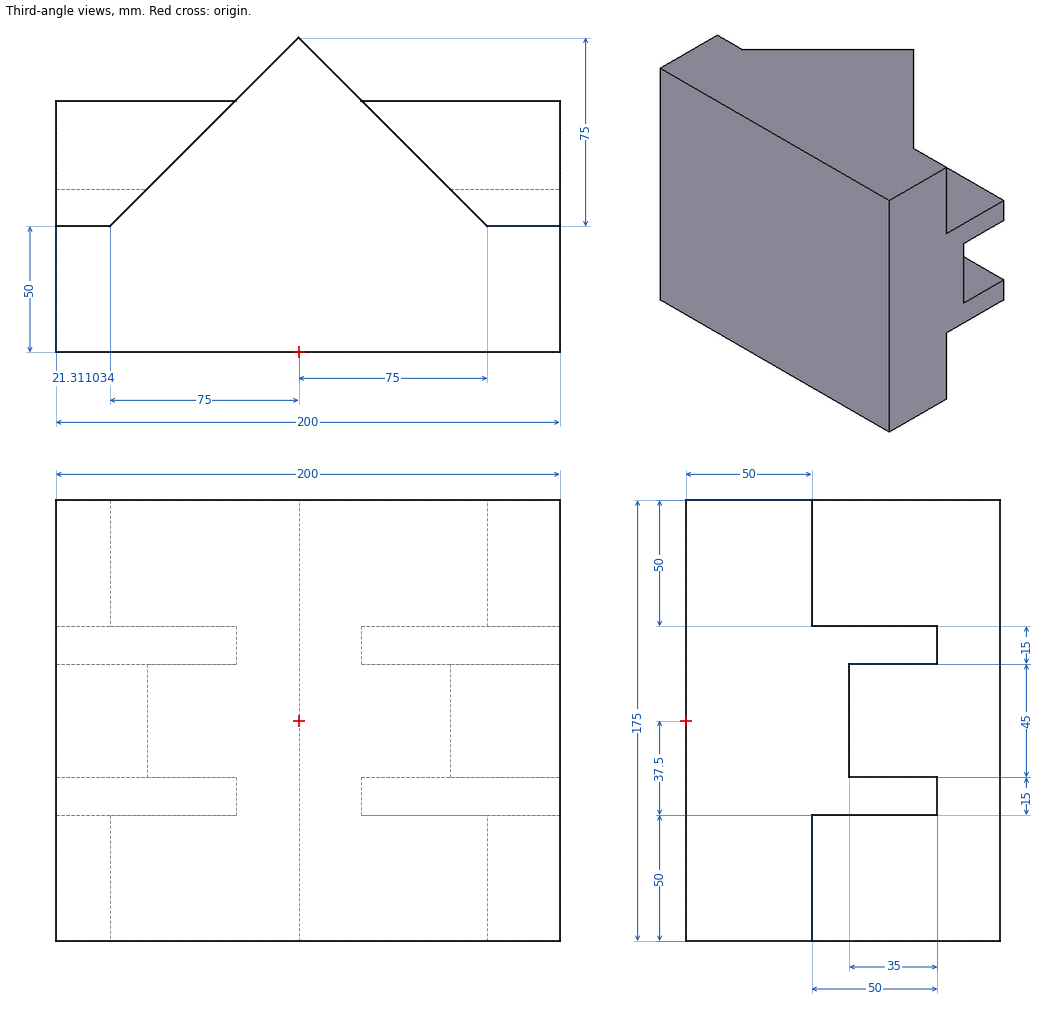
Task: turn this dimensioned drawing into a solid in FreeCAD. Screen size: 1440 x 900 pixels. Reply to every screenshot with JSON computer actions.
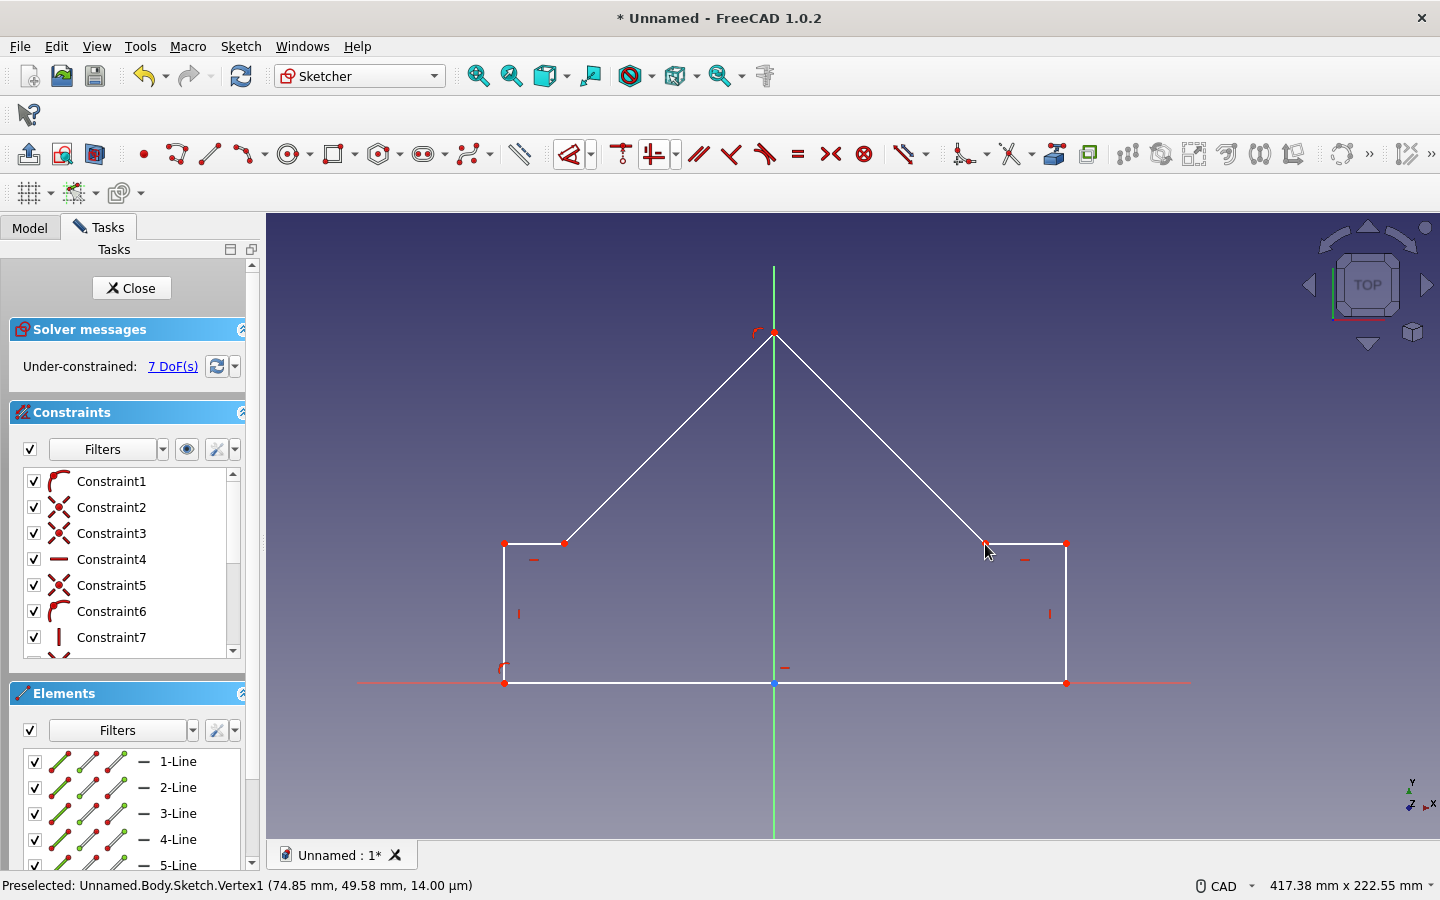
{"action": "left_click", "coordinate": [568, 154]}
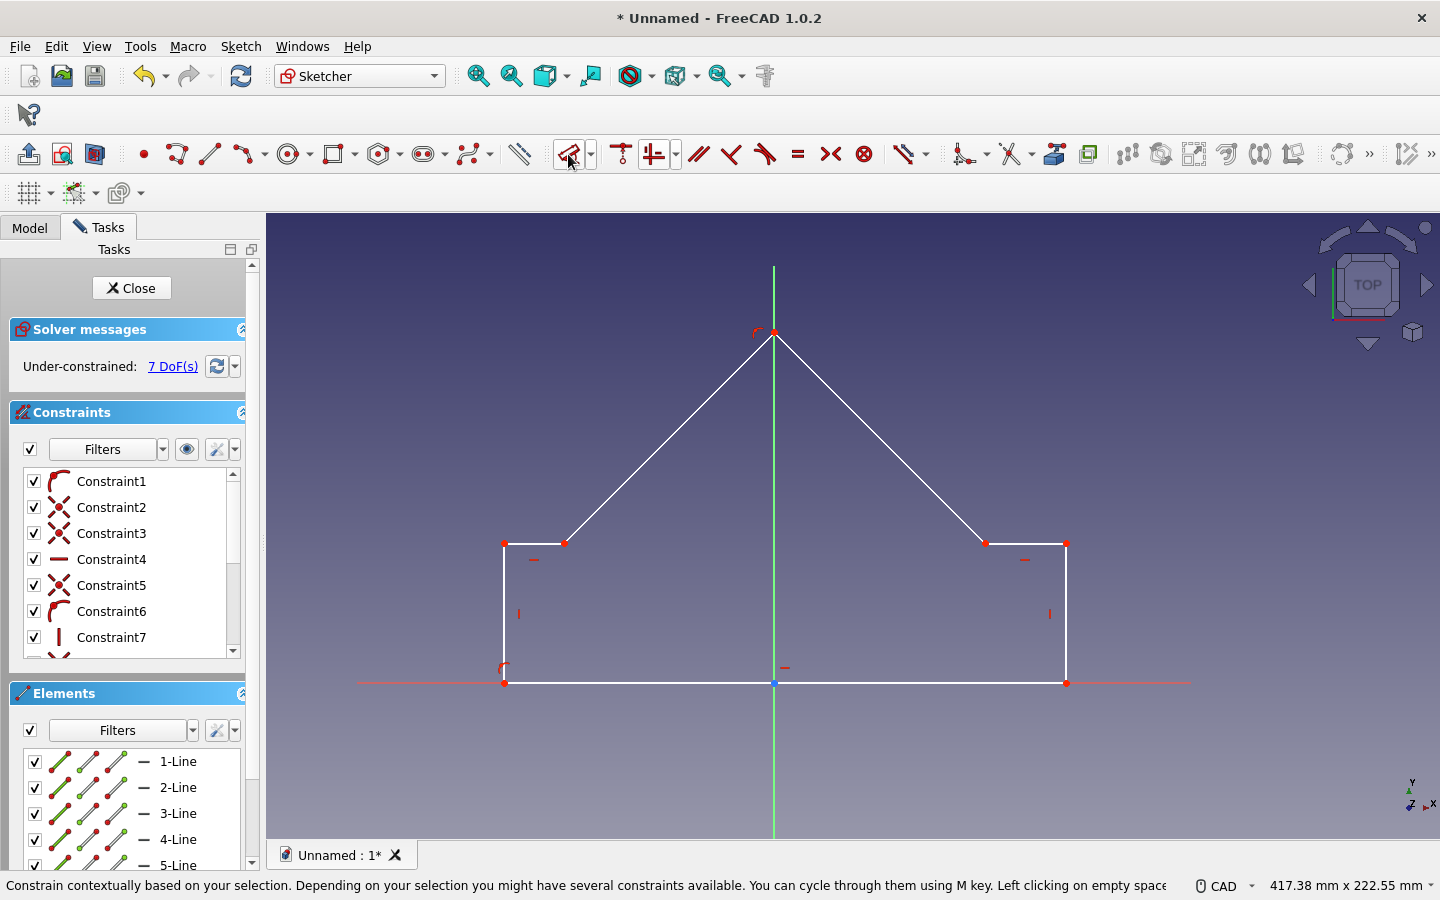
{"action": "left_click", "coordinate": [504, 586]}
{"action": "left_click", "coordinate": [470, 614]}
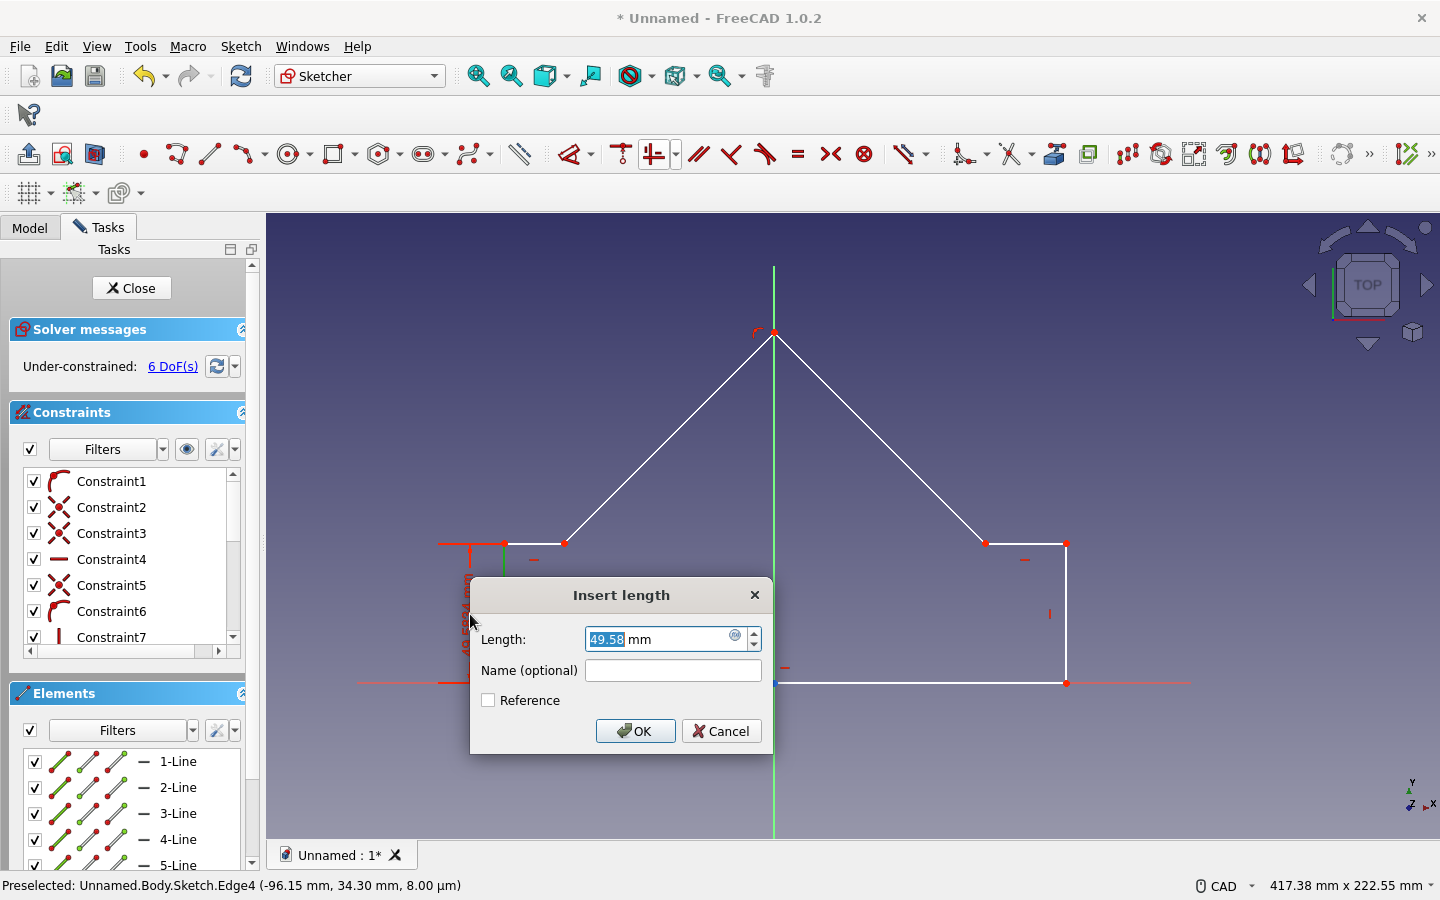
{"action": "type", "text": "50"}
{"action": "key", "text": "Return"}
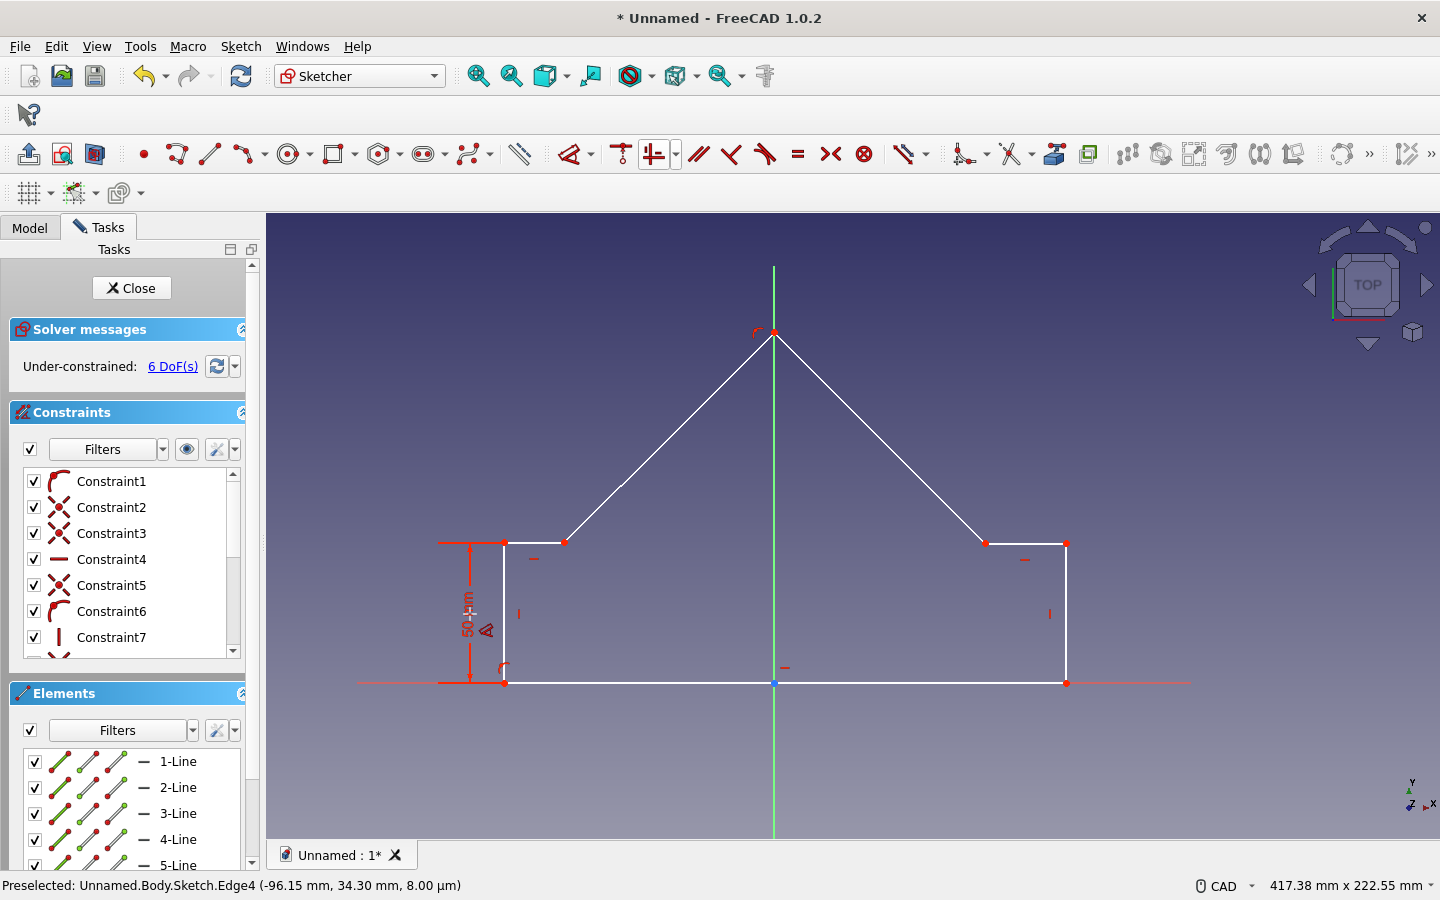
{"action": "left_click", "coordinate": [1066, 642]}
{"action": "left_click", "coordinate": [1100, 614]}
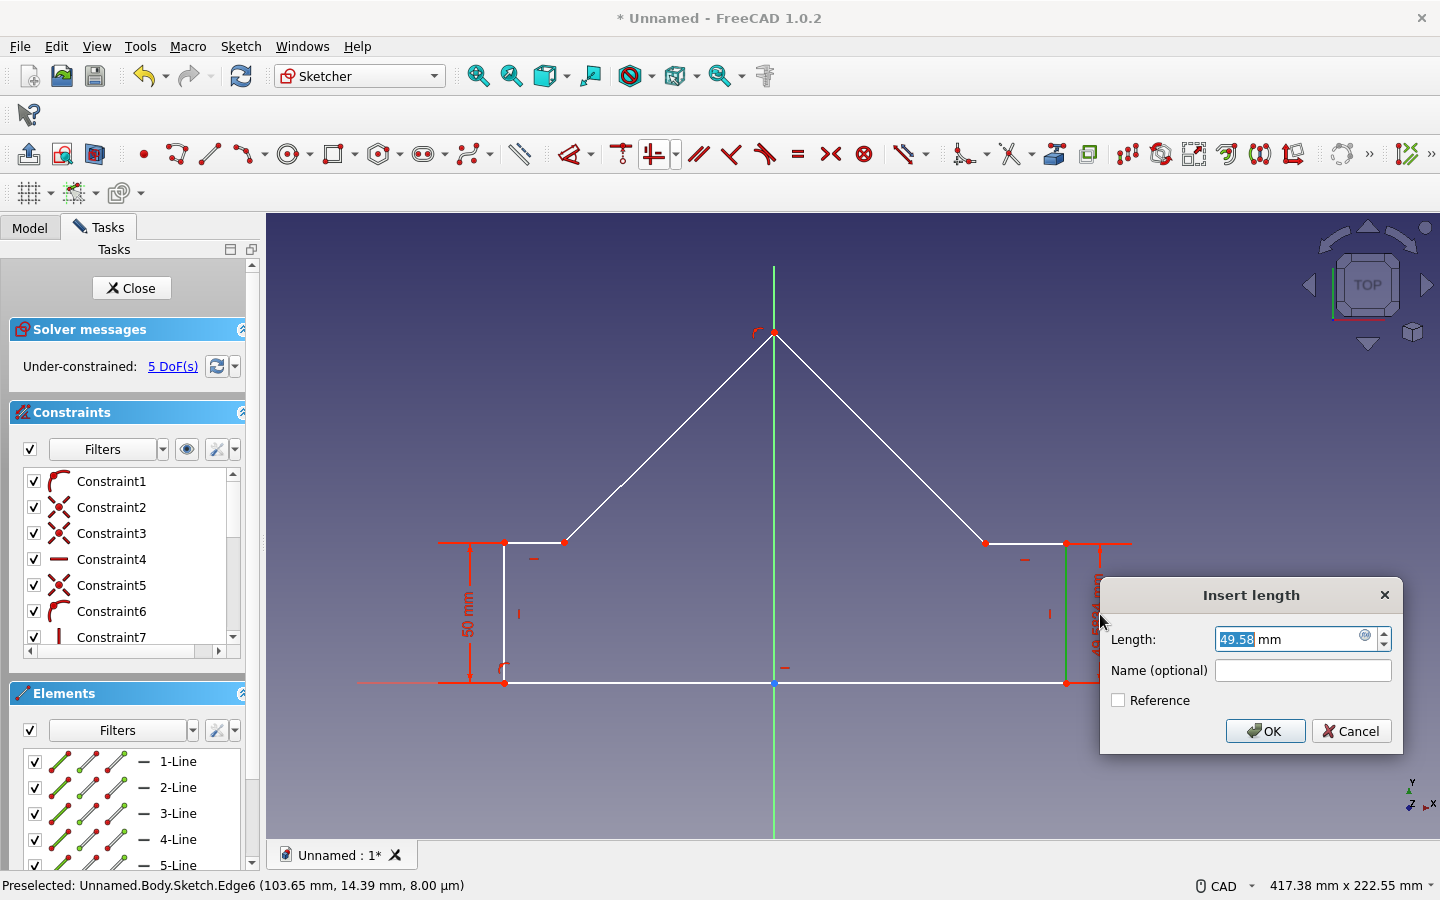
{"action": "type", "text": "50"}
{"action": "key", "text": "Return"}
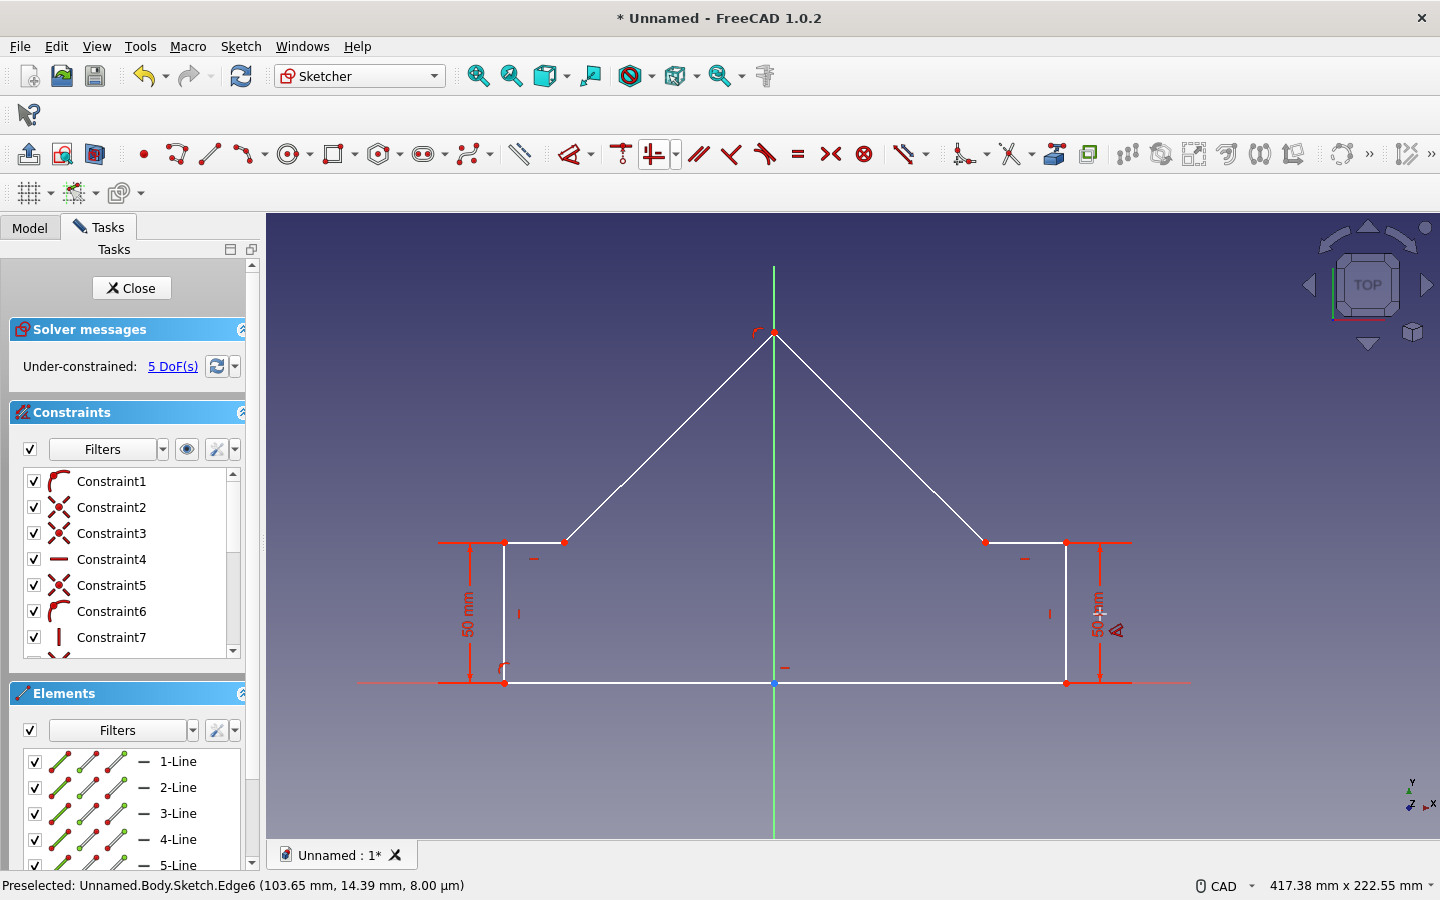
{"action": "left_click", "coordinate": [673, 683]}
{"action": "left_click", "coordinate": [656, 717]}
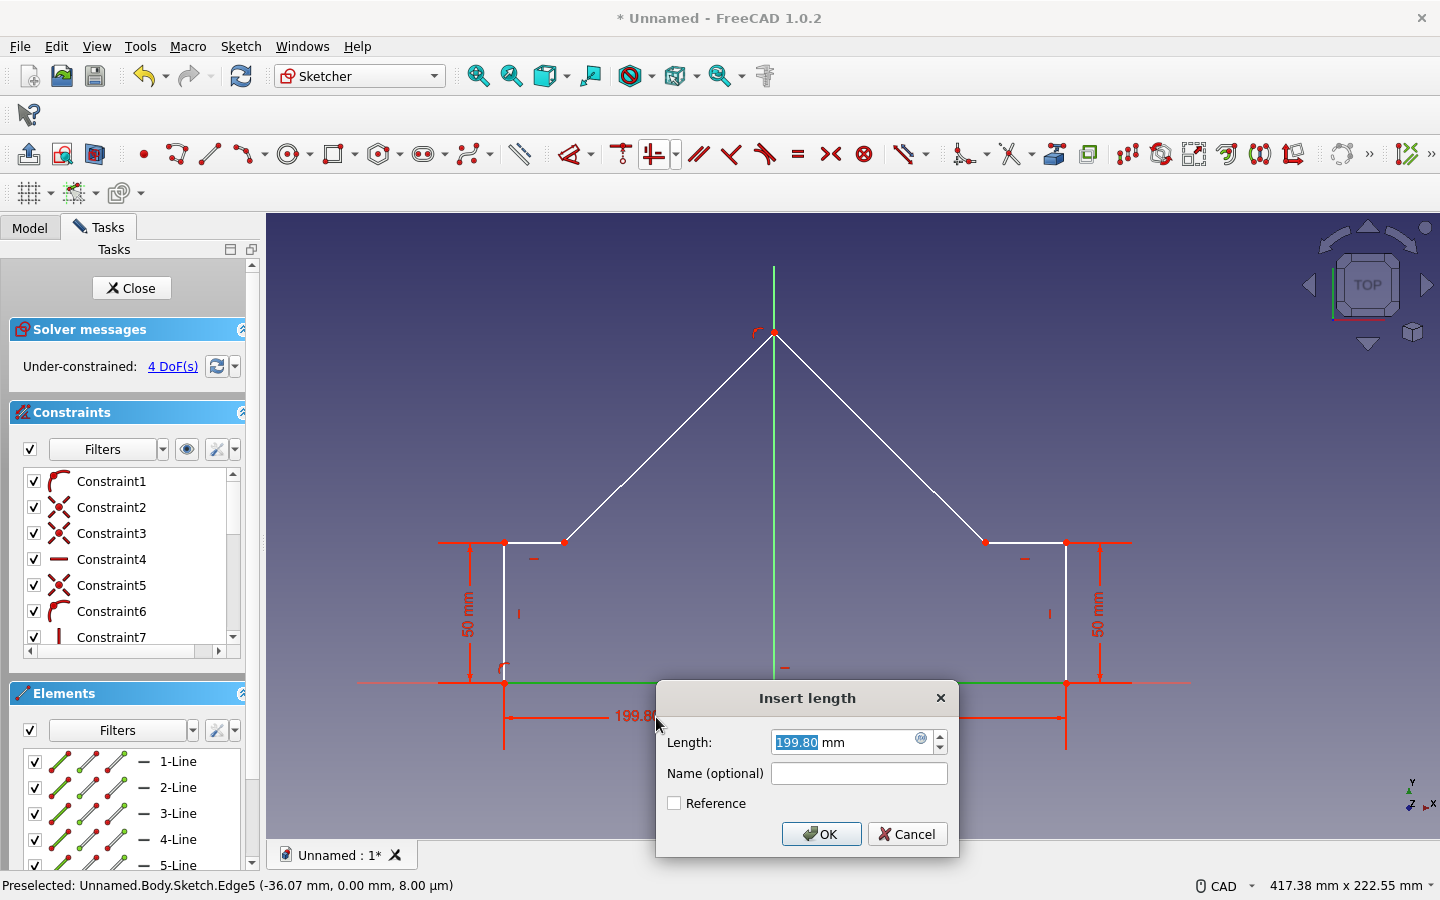
{"action": "type", "text": "200"}
{"action": "key", "text": "Return"}